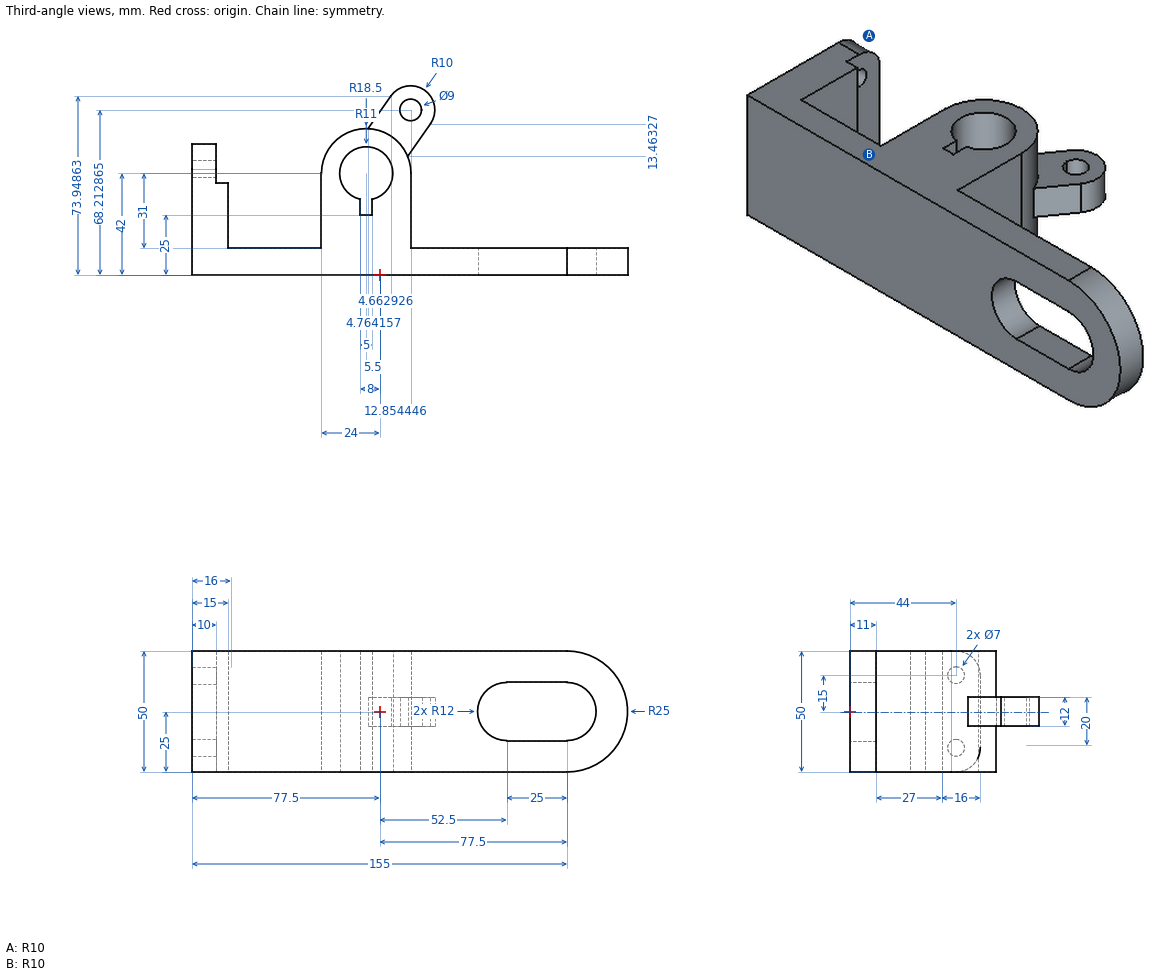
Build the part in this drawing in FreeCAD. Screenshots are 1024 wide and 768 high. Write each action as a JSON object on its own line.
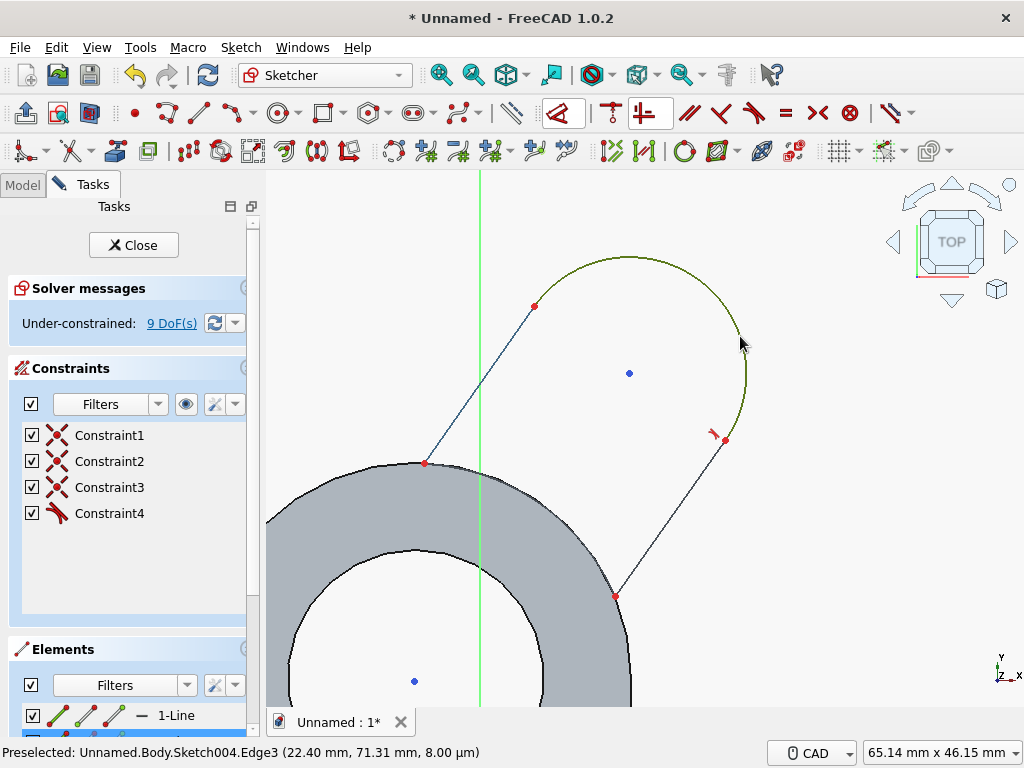
{"action": "key", "text": "t"}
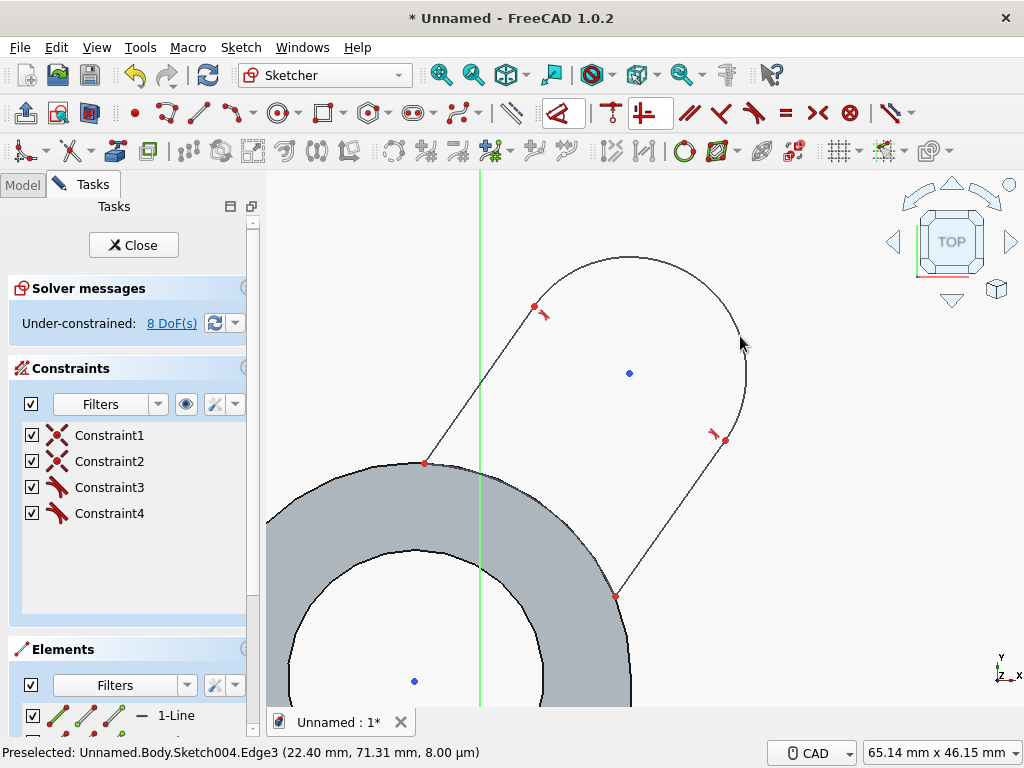
{"action": "left_click", "coordinate": [740, 336]}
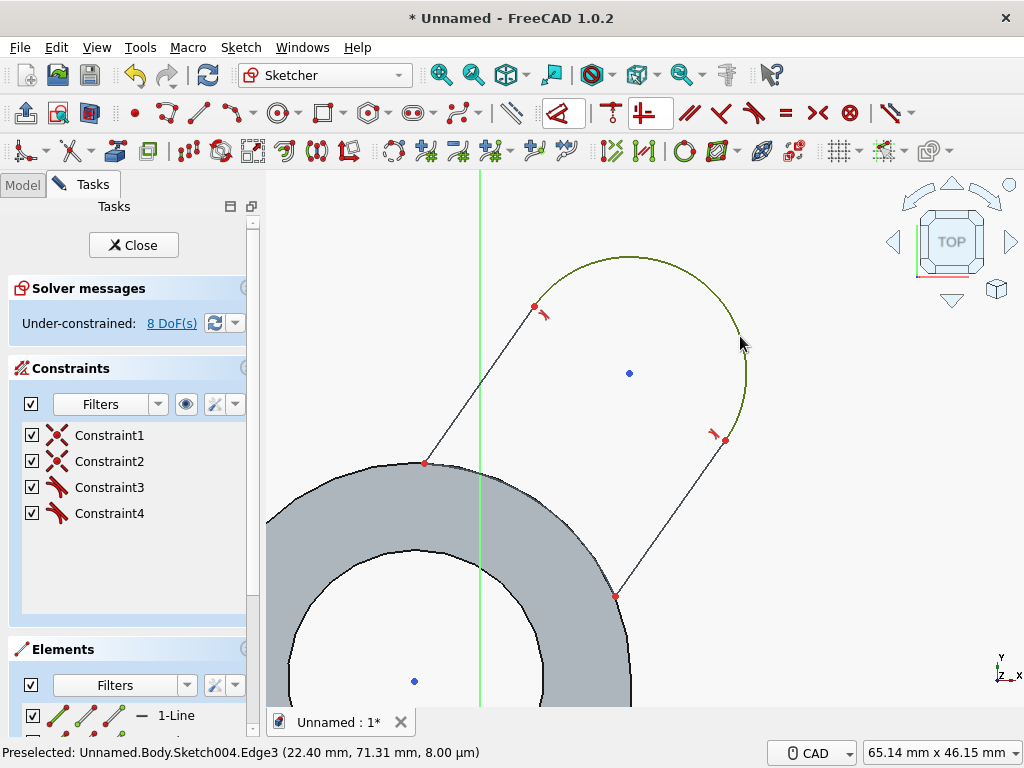
{"action": "key", "text": "k r"}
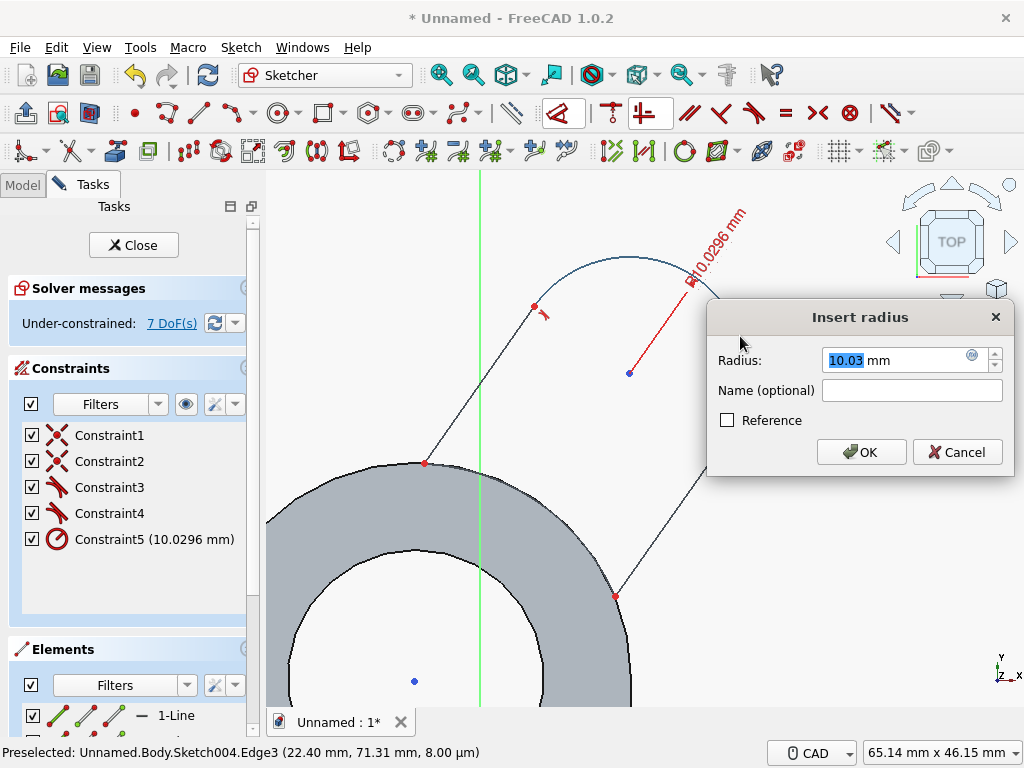
{"action": "type", "text": "10"}
{"action": "key", "text": "Return"}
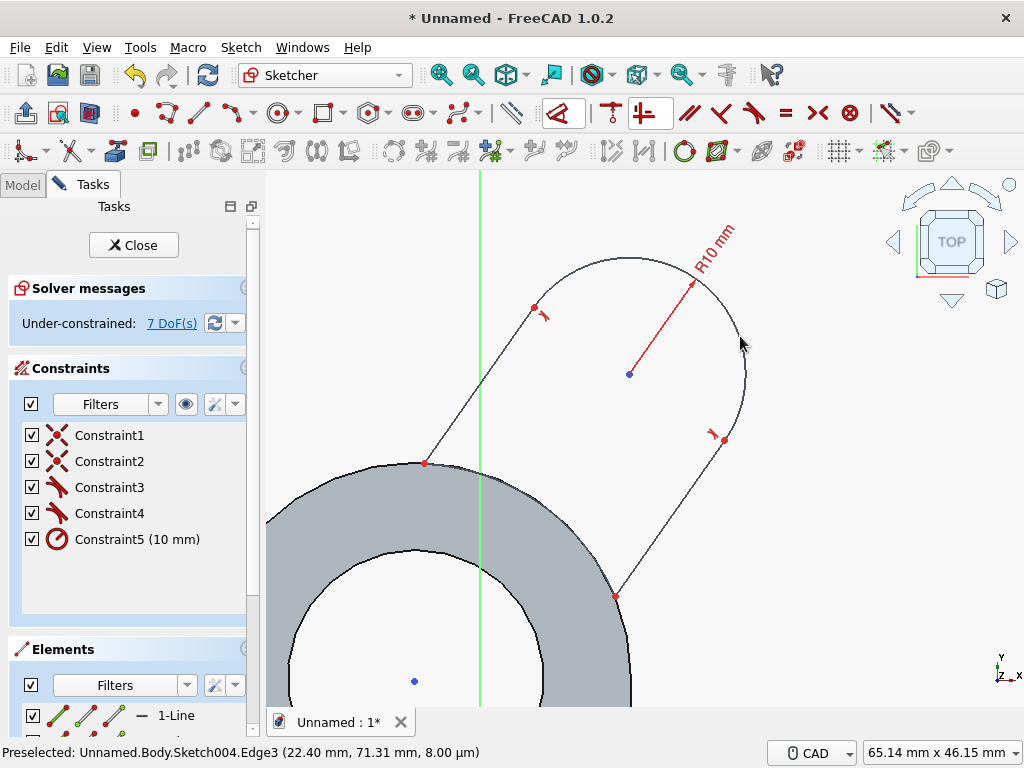
{"action": "left_click", "coordinate": [576, 535]}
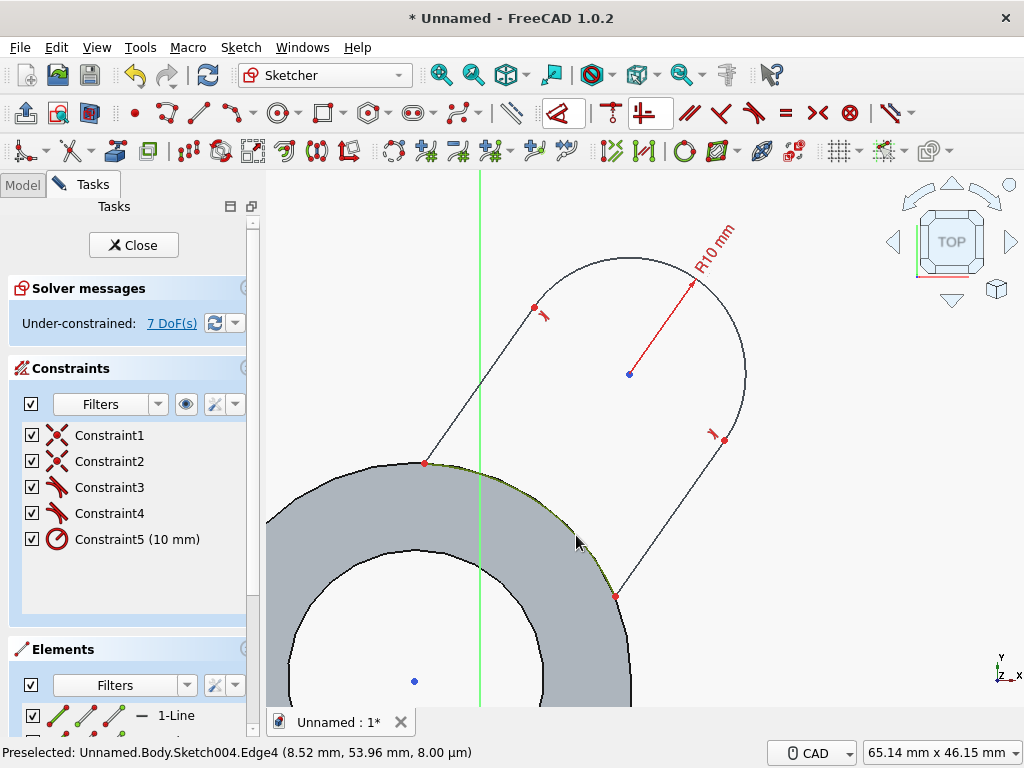
{"action": "key", "text": "k r"}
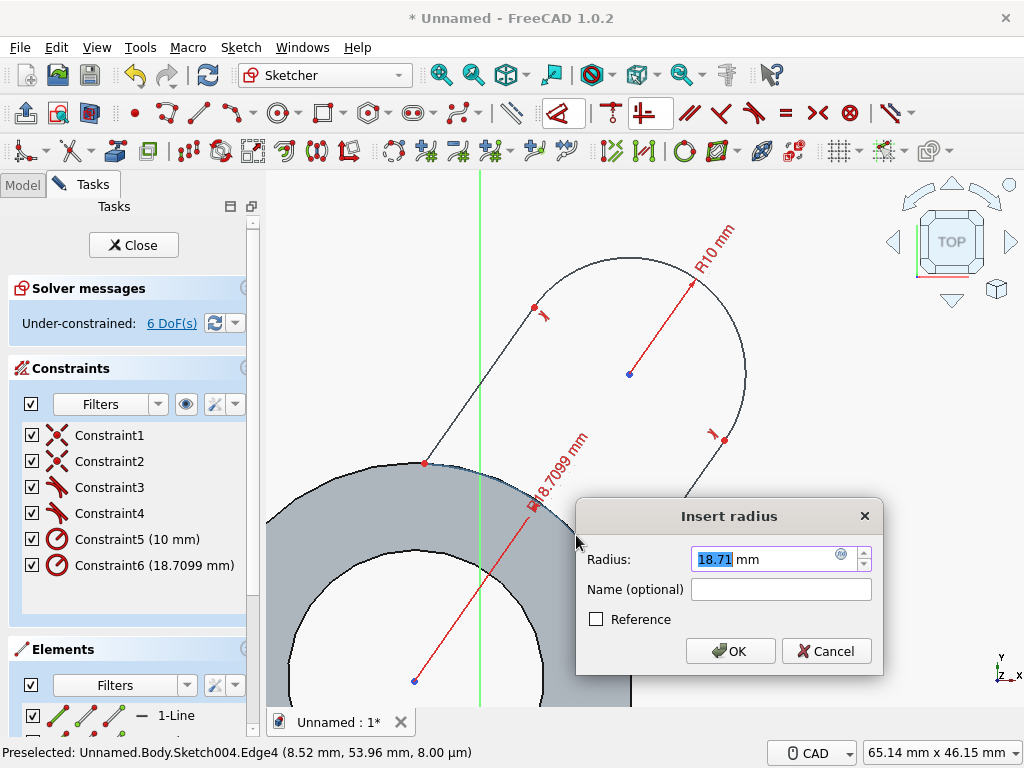
{"action": "type", "text": "18.5"}
{"action": "key", "text": "Return"}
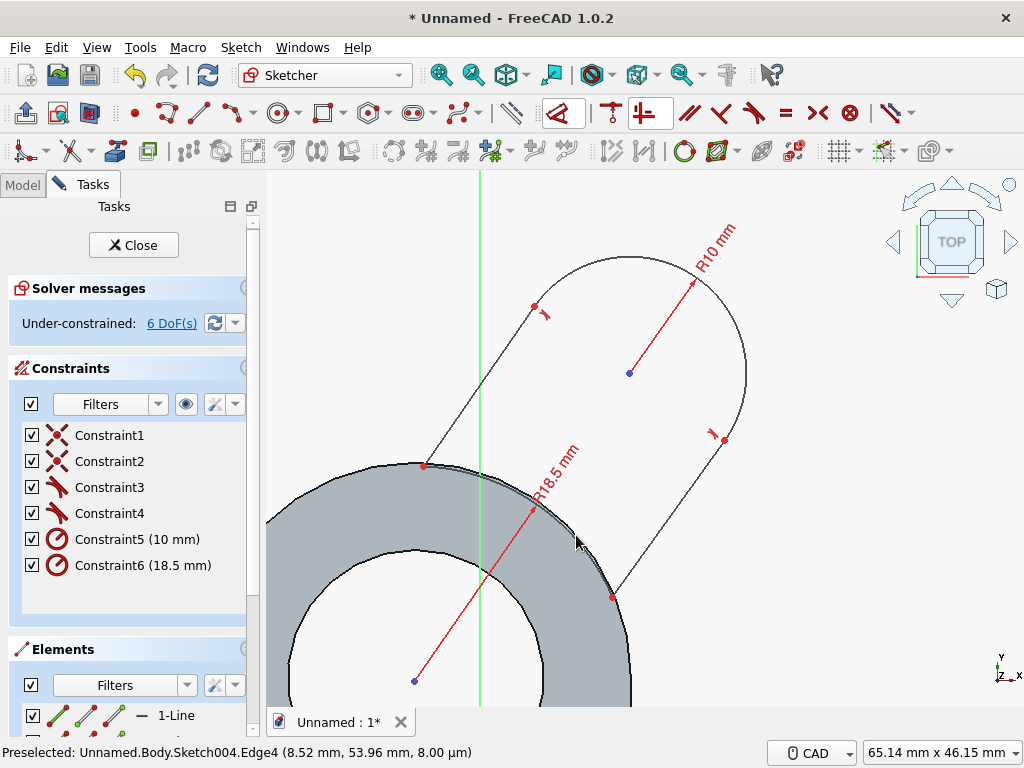
{"action": "scroll", "coordinate": [608, 253], "scroll_direction": "down", "scroll_amount": 1}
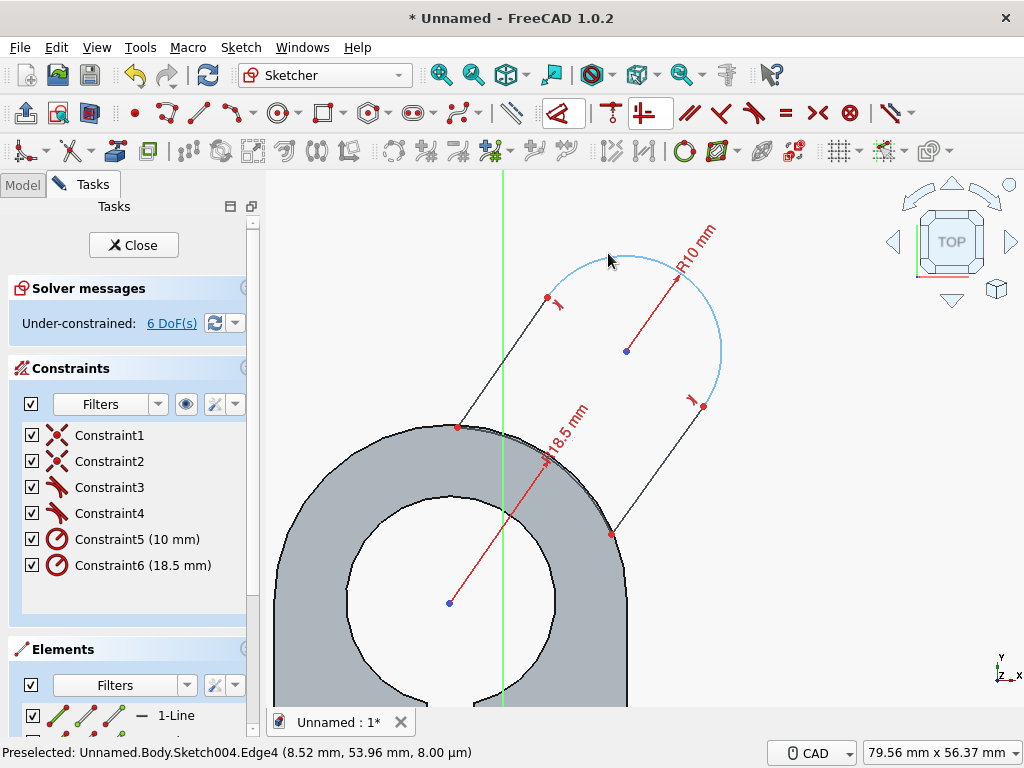
{"action": "left_click", "coordinate": [450, 604]}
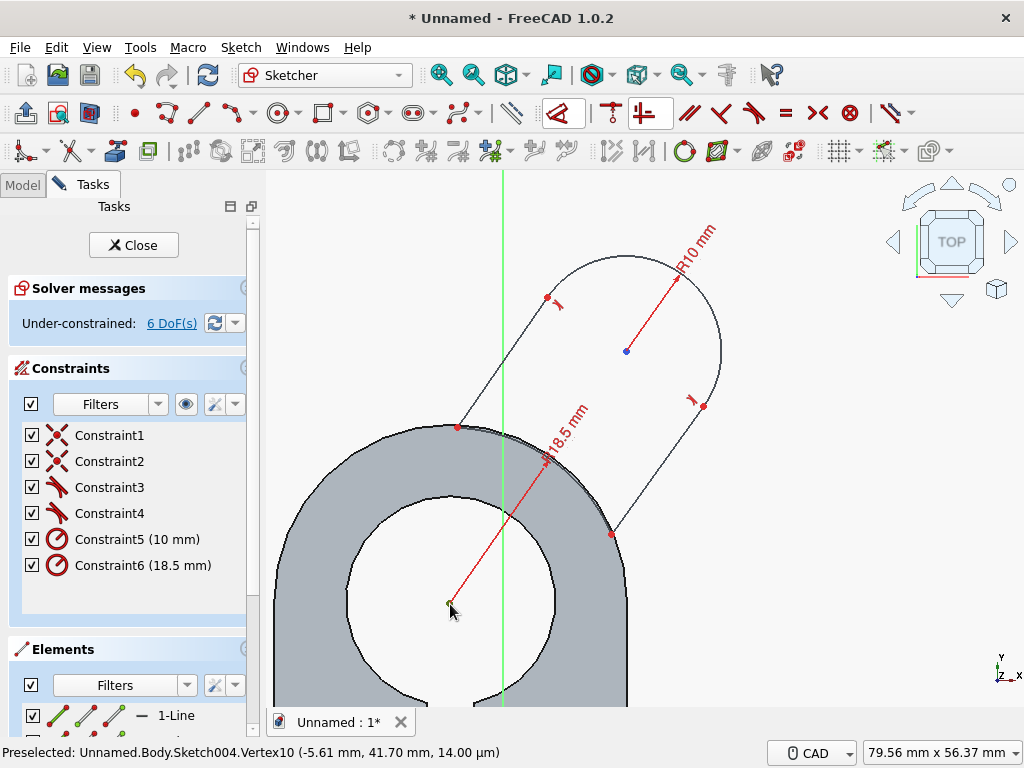
{"action": "left_click", "coordinate": [580, 114]}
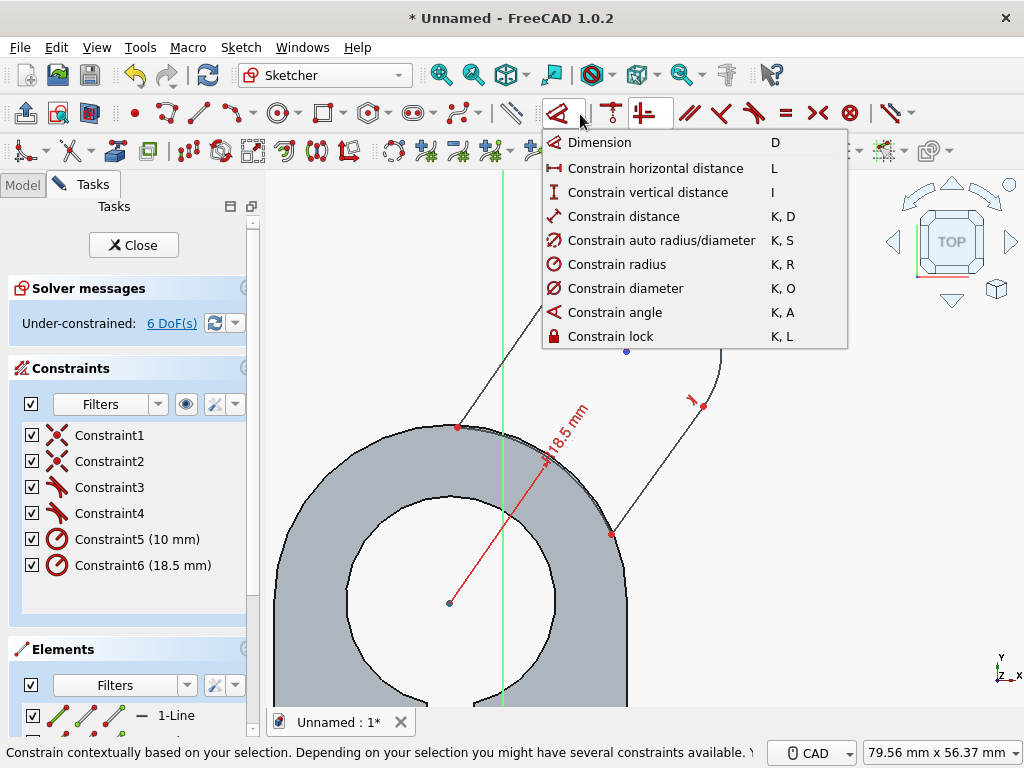
{"action": "left_click", "coordinate": [695, 192]}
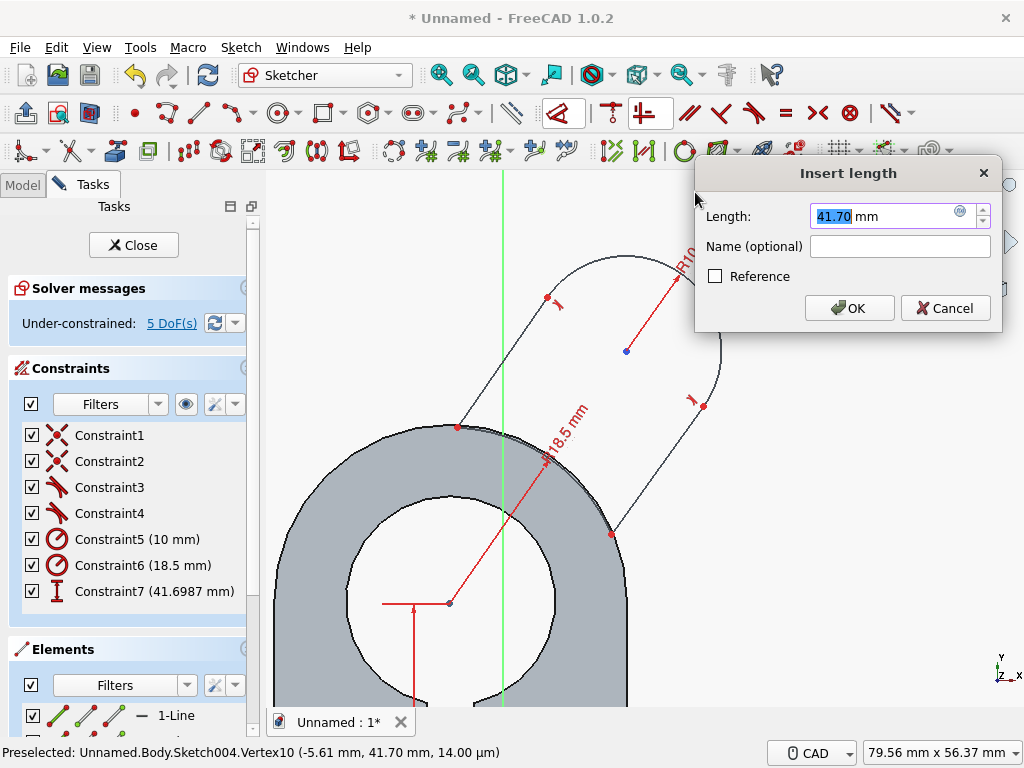
{"action": "type", "text": "42"}
{"action": "key", "text": "Return"}